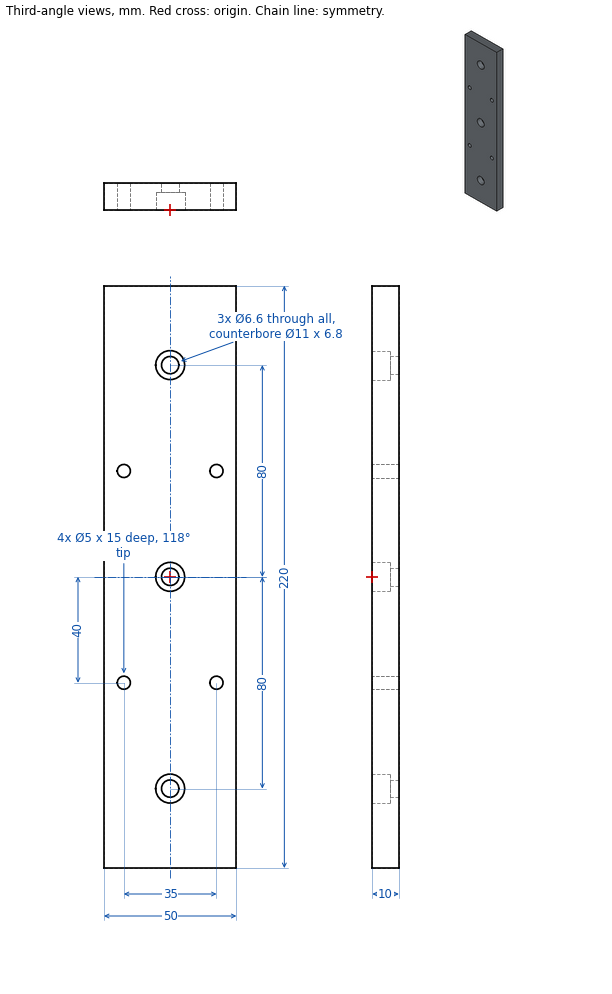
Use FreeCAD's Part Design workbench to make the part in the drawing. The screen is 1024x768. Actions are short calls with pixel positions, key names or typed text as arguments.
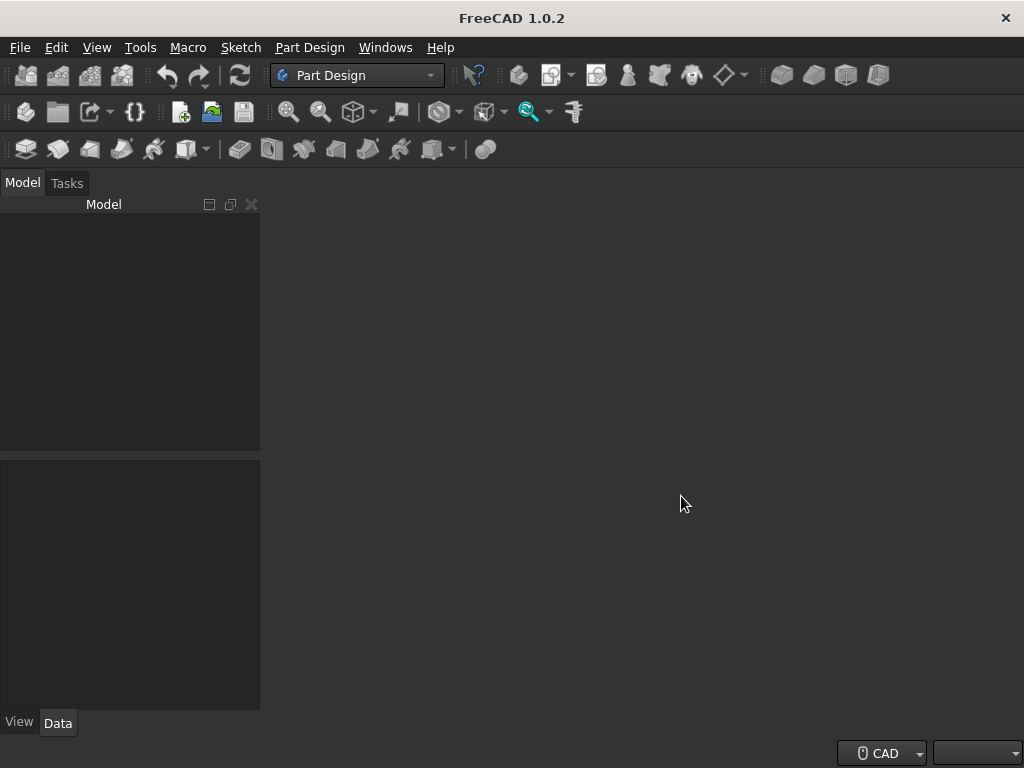
click(180, 112)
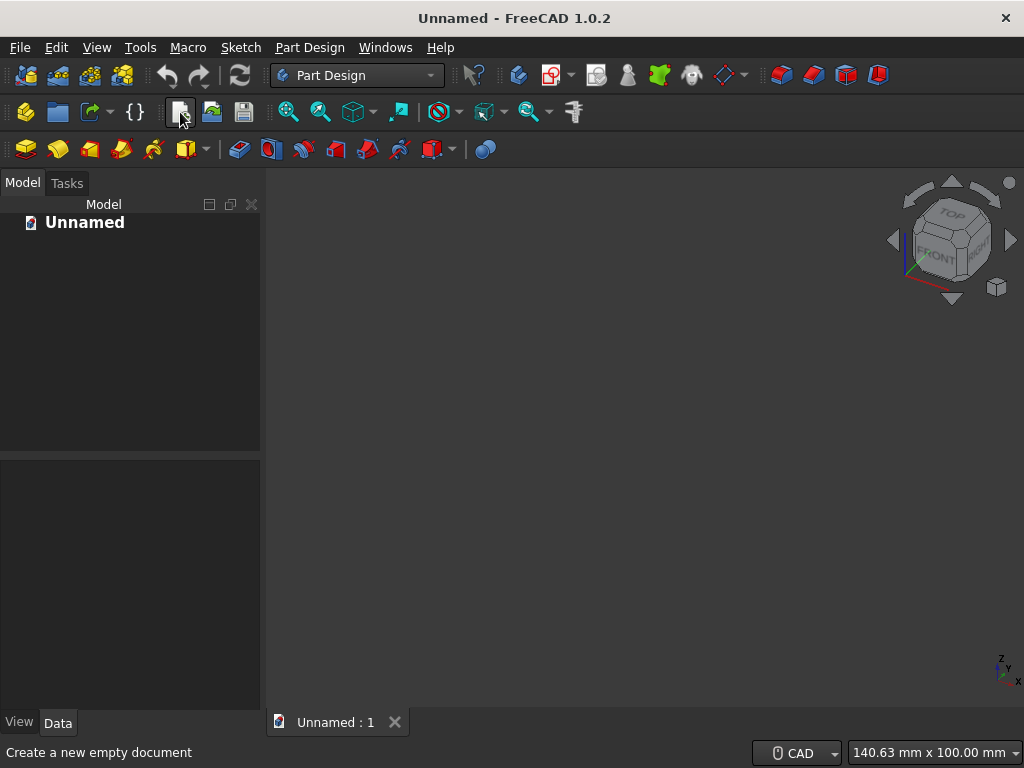
click(552, 76)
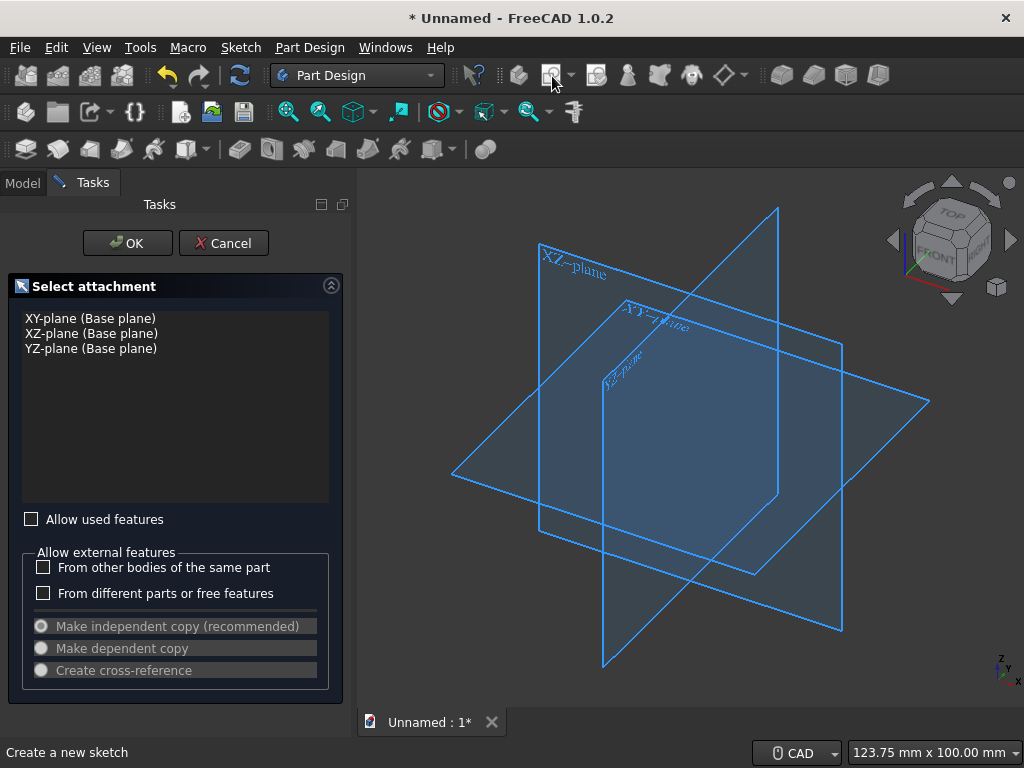
click(82, 334)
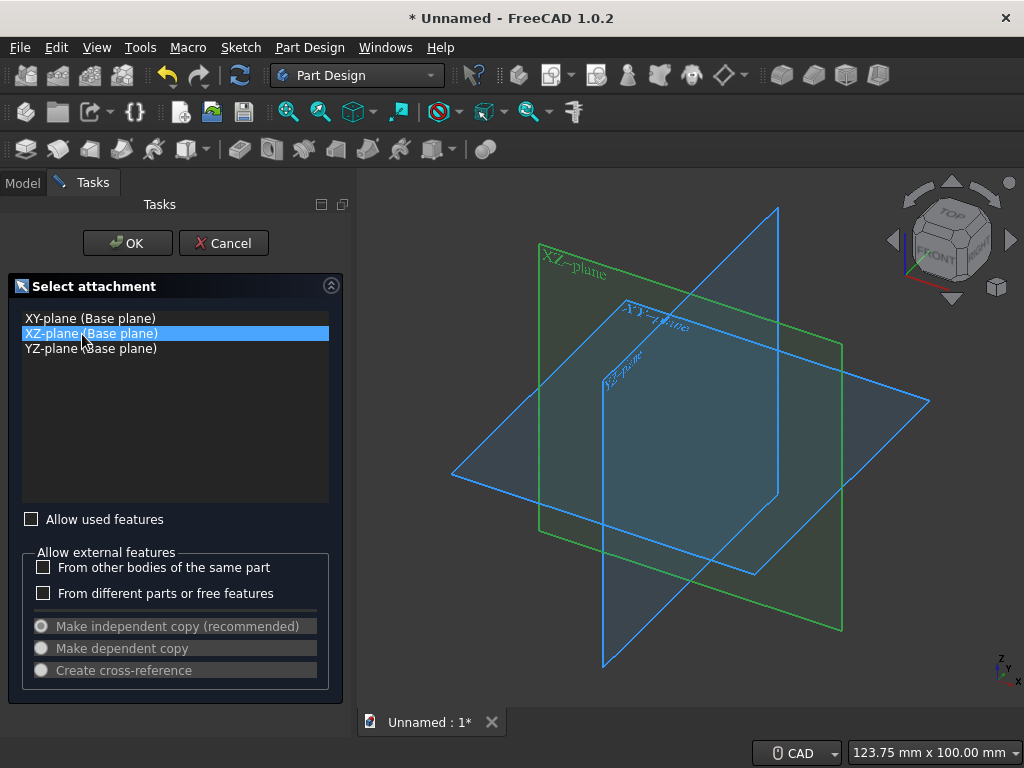
click(128, 243)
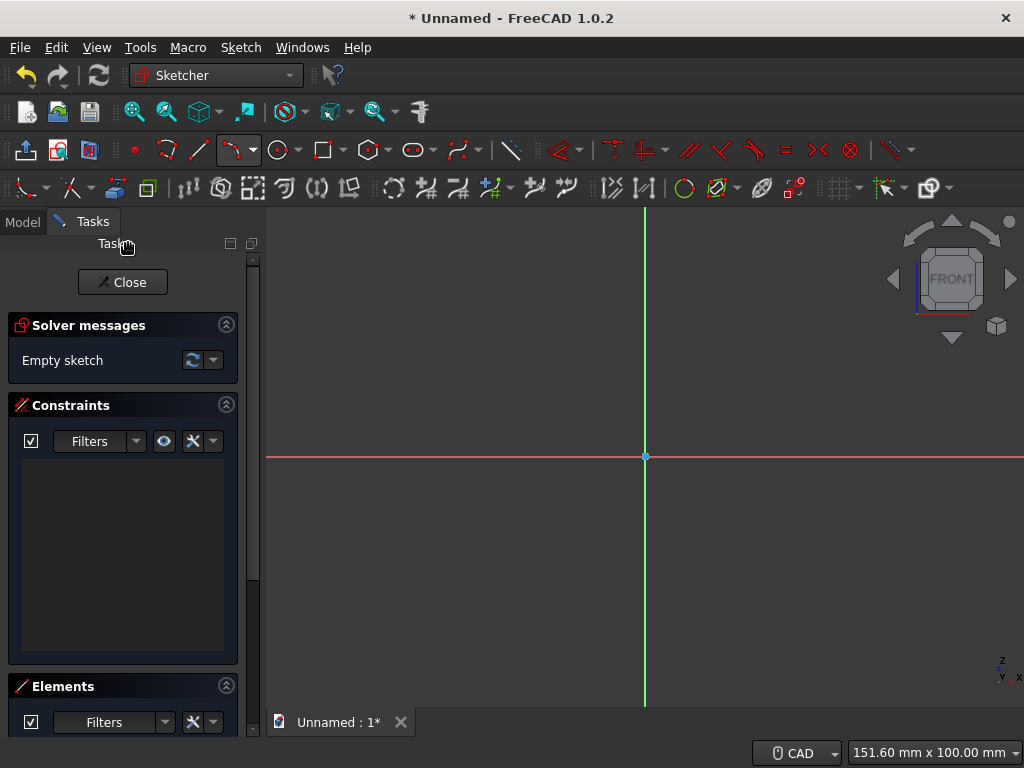
scroll(547, 457, down, 6)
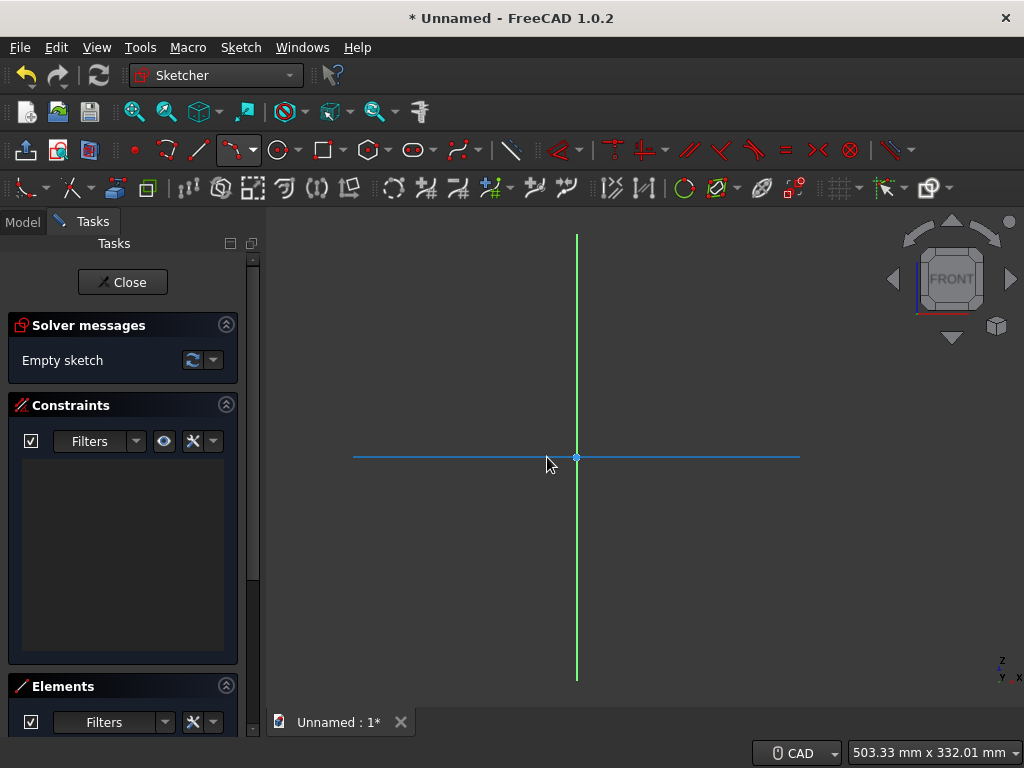
click(346, 150)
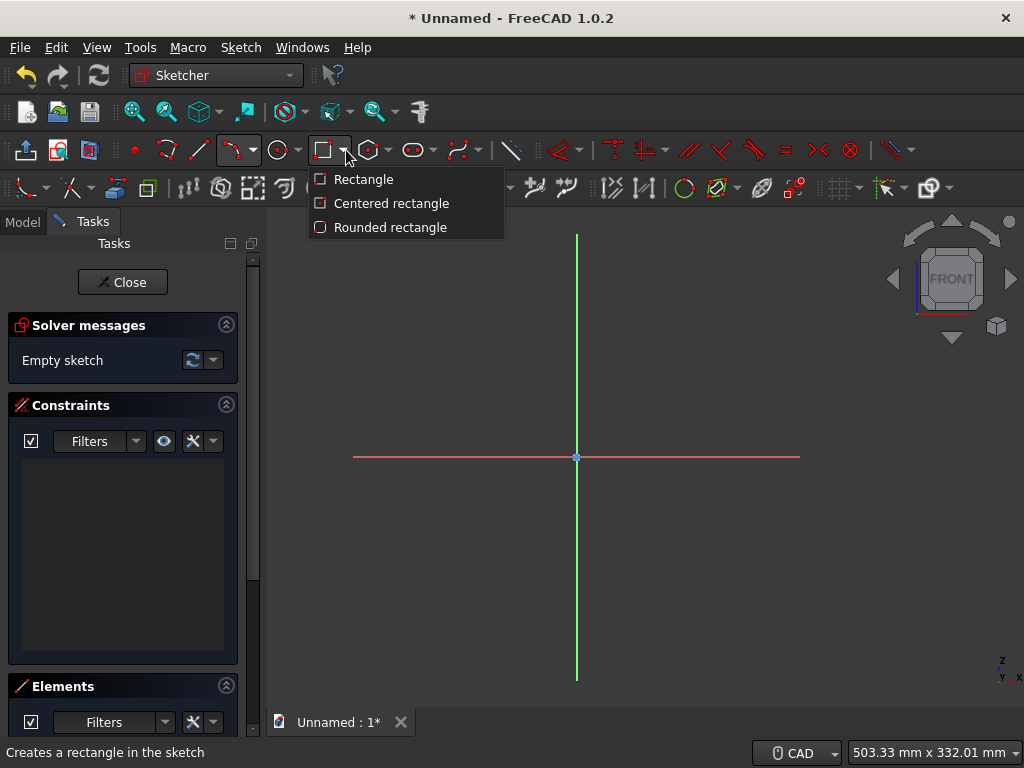
click(406, 203)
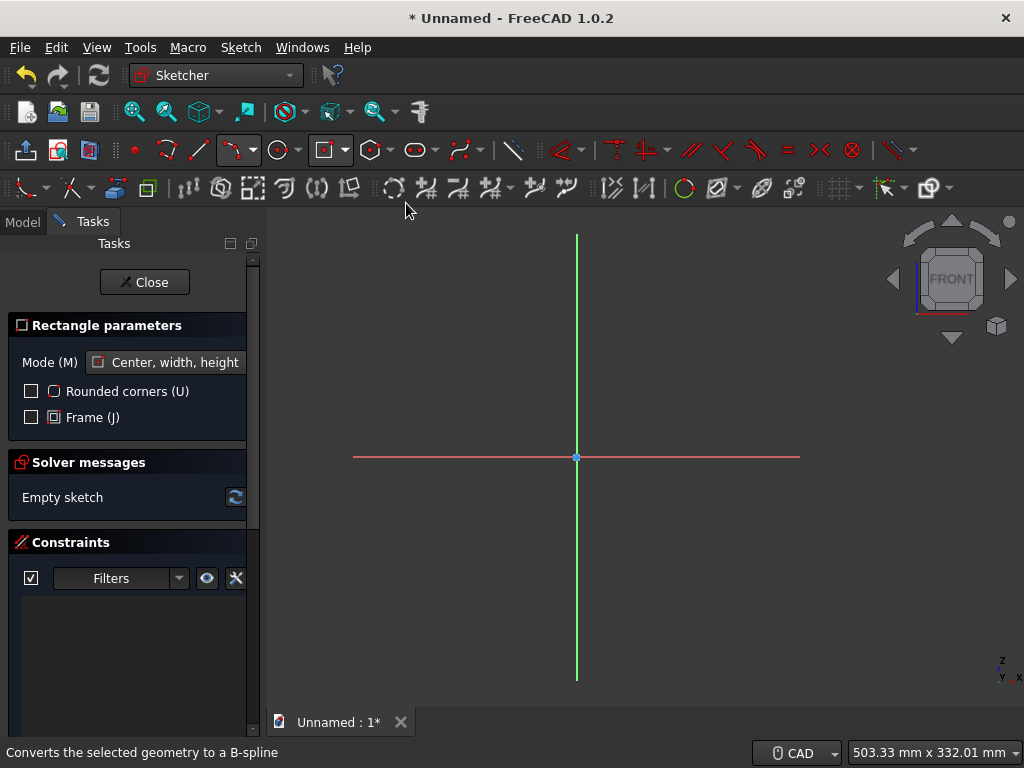
click(577, 457)
move(614, 292)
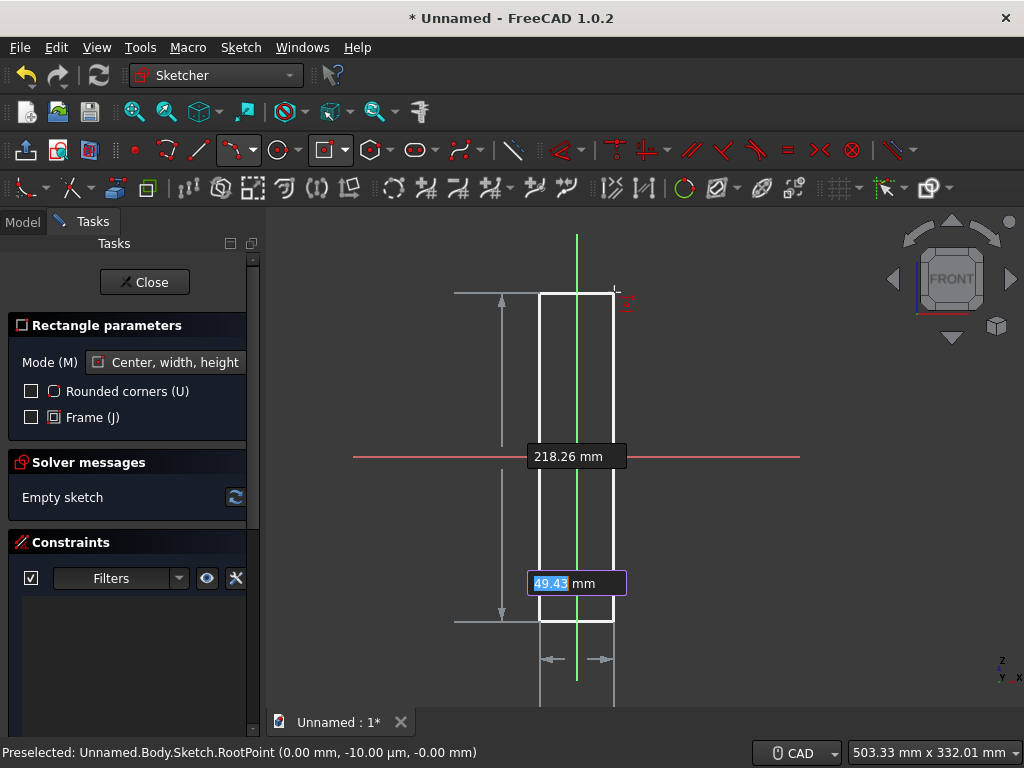
text(50)
key(Tab)
text(220)
key(Return)
key(Escape)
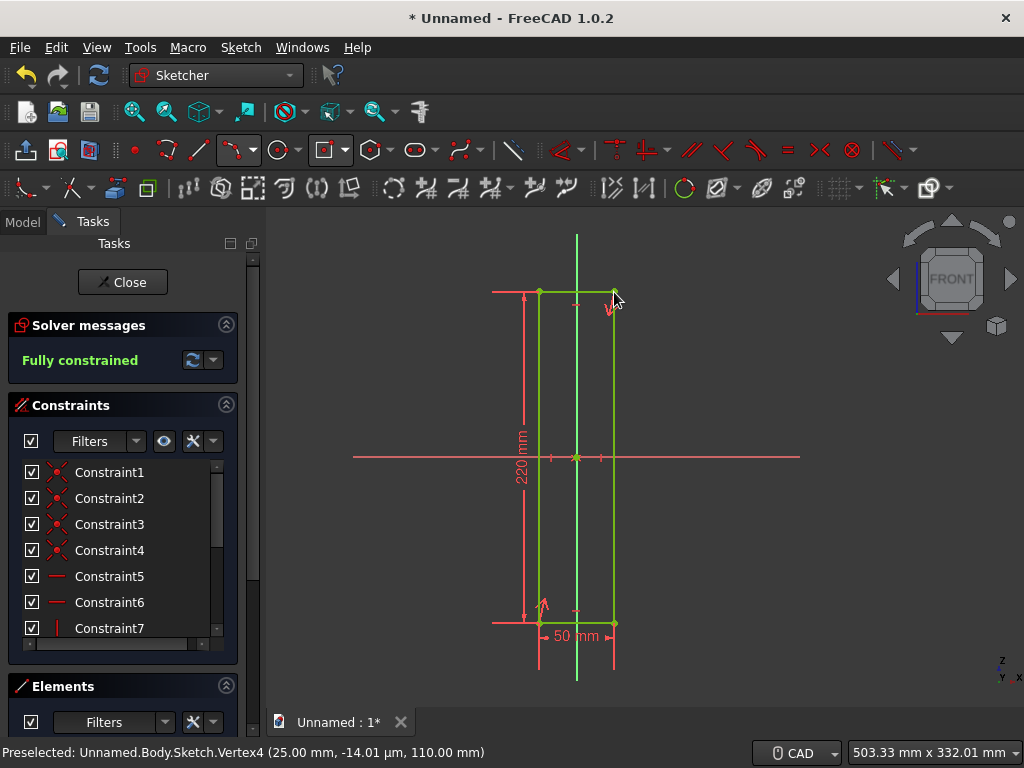
click(123, 282)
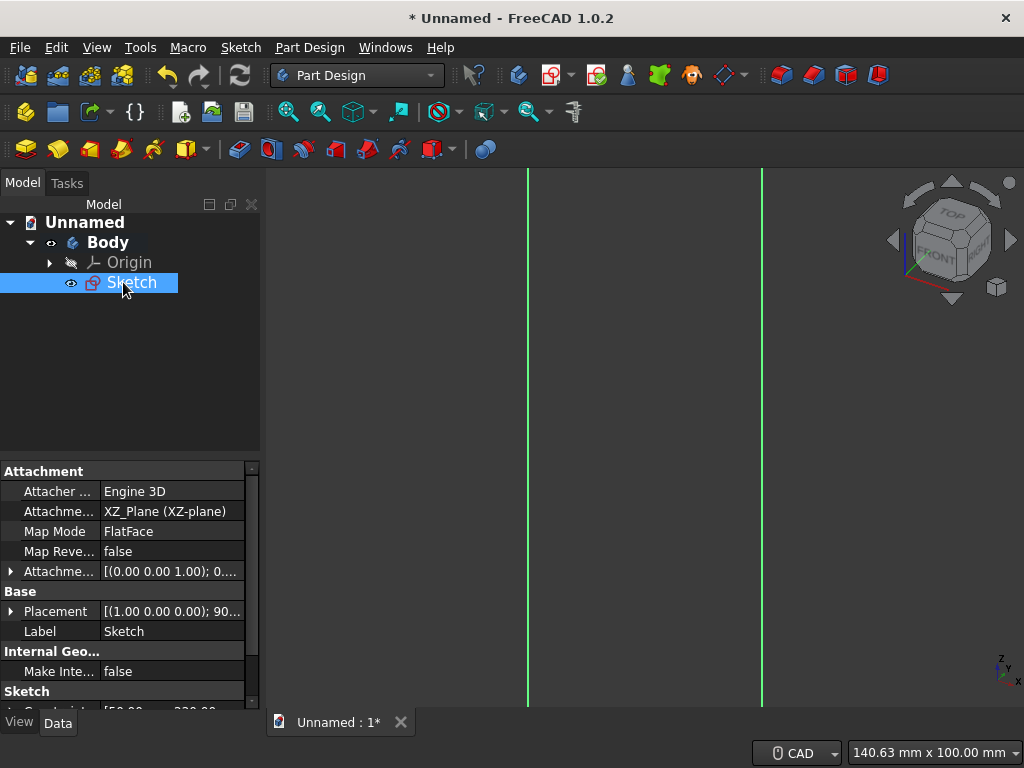
click(26, 150)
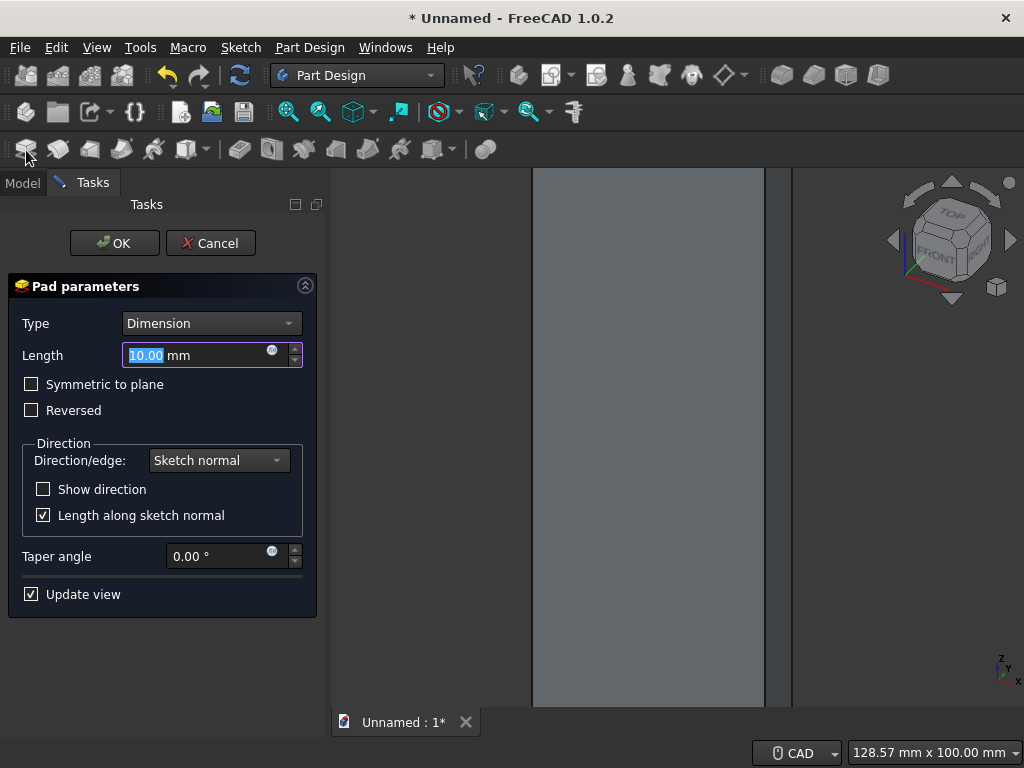
text(10)
key(Tab)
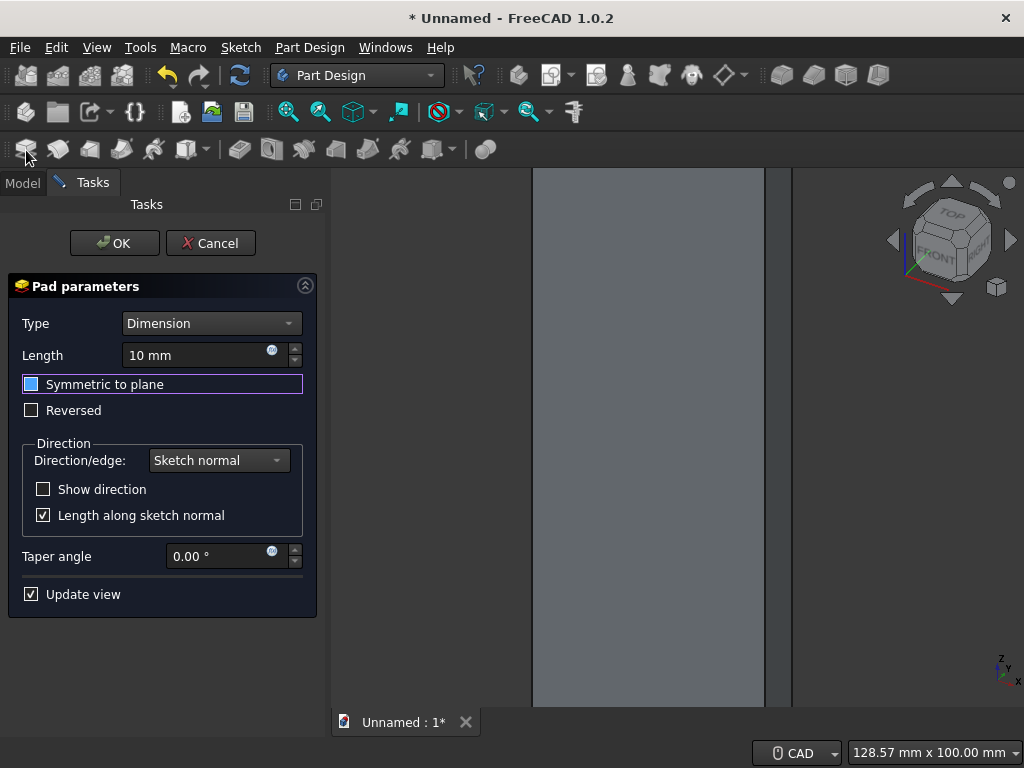
click(30, 410)